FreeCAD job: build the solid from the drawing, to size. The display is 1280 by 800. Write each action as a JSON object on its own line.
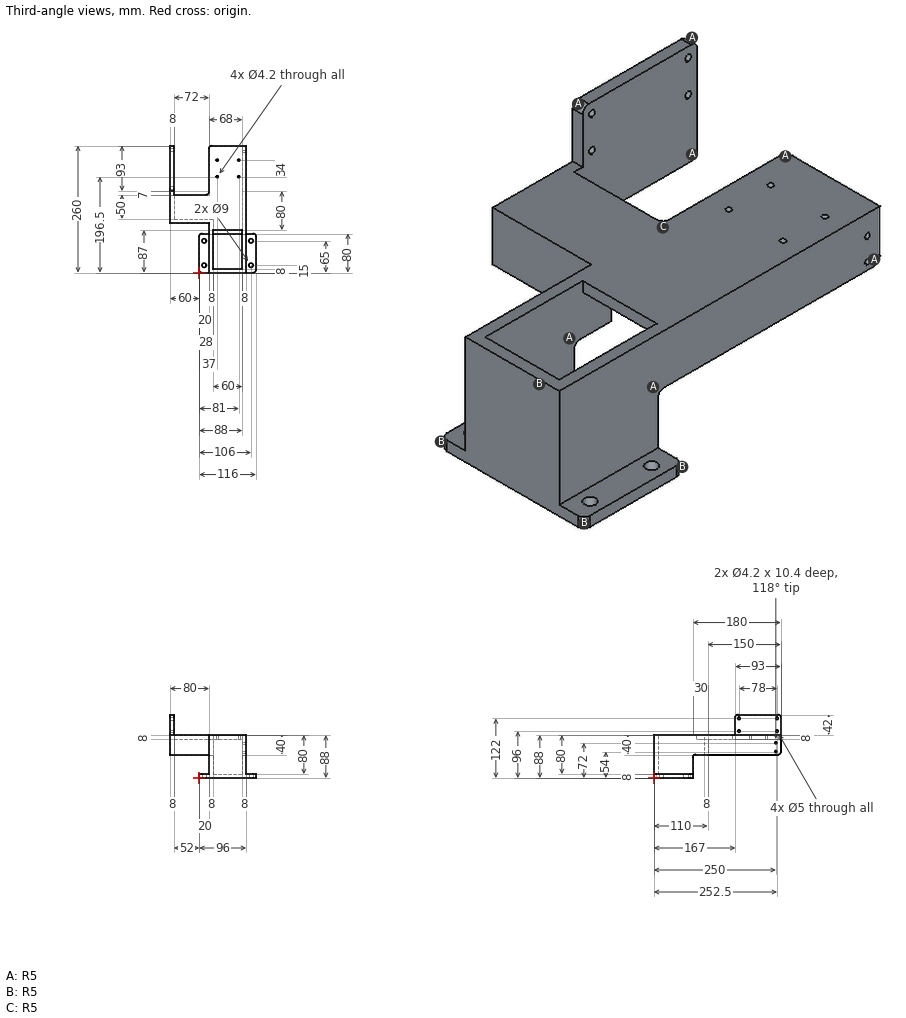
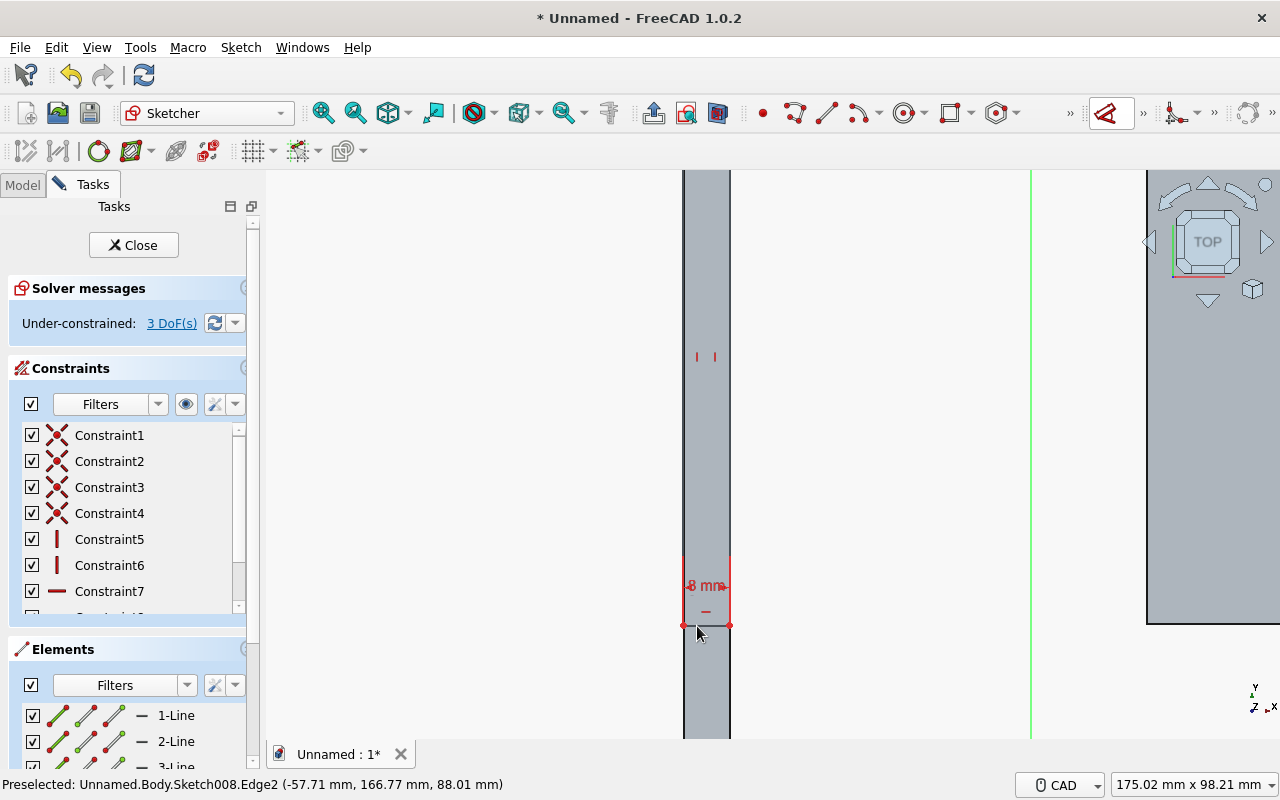
{"action": "left_click", "coordinate": [683, 249]}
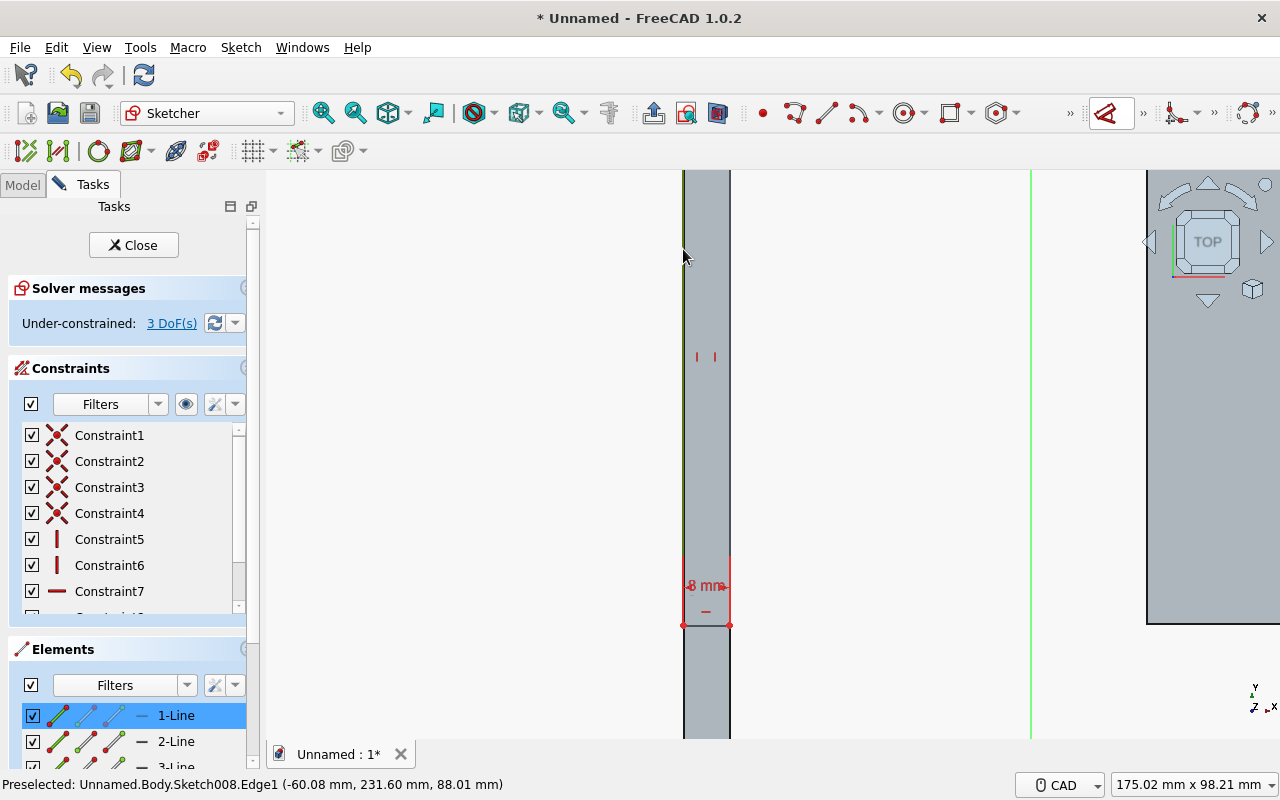
{"action": "left_click", "coordinate": [1128, 114]}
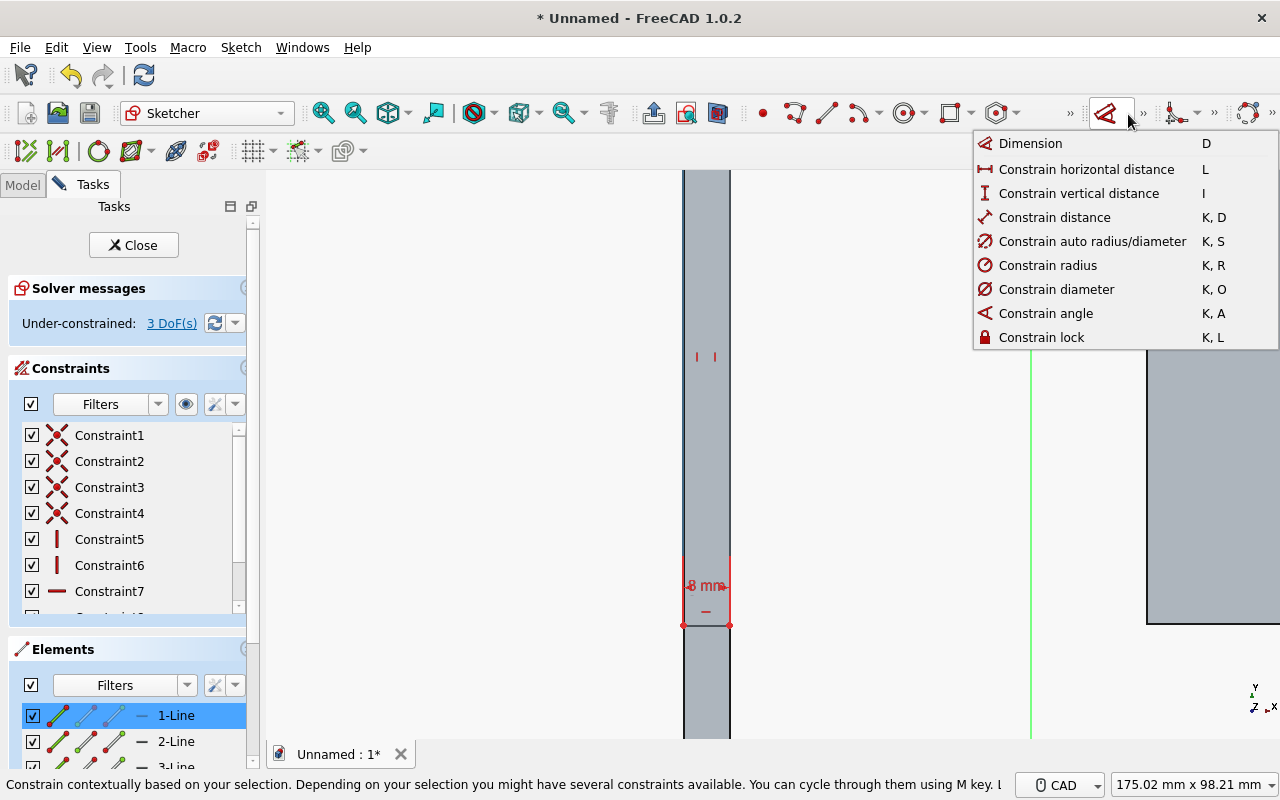
{"action": "left_click", "coordinate": [1126, 193]}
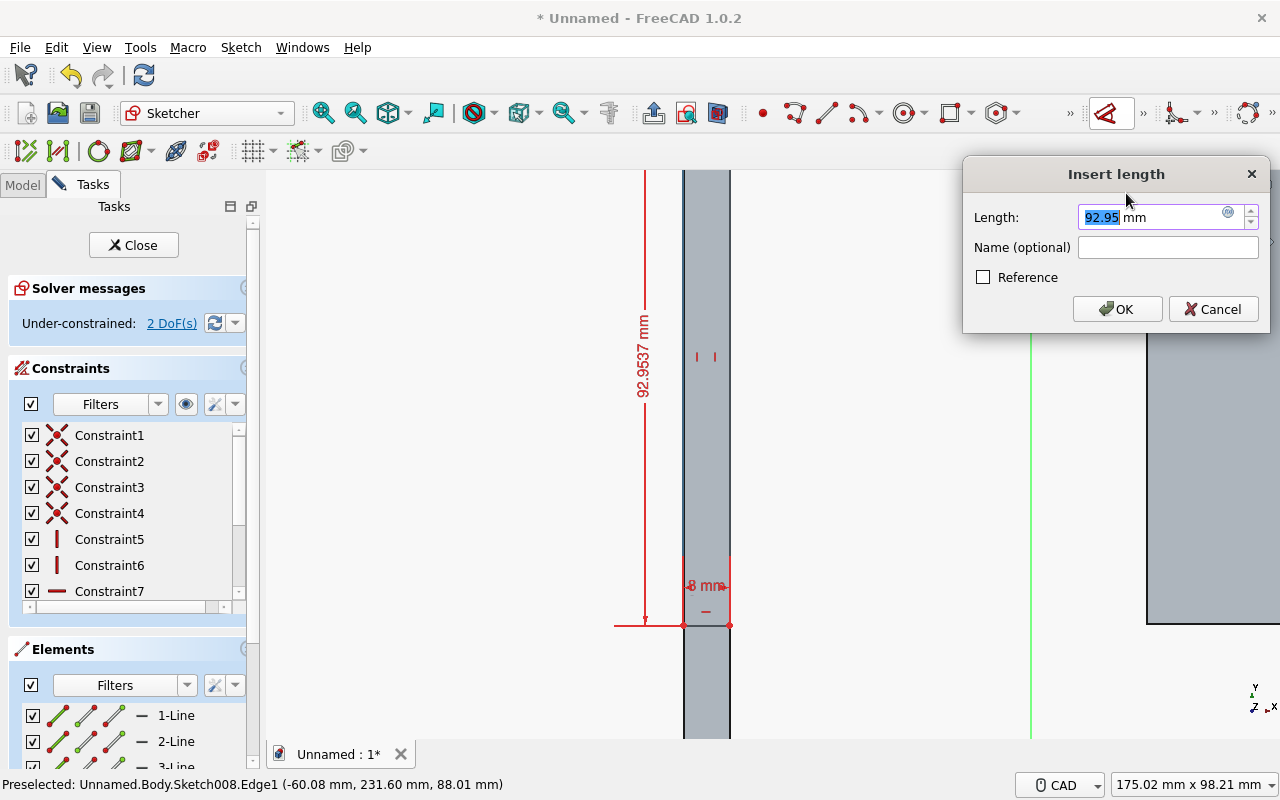
{"action": "type", "text": "93"}
{"action": "key", "text": "Return"}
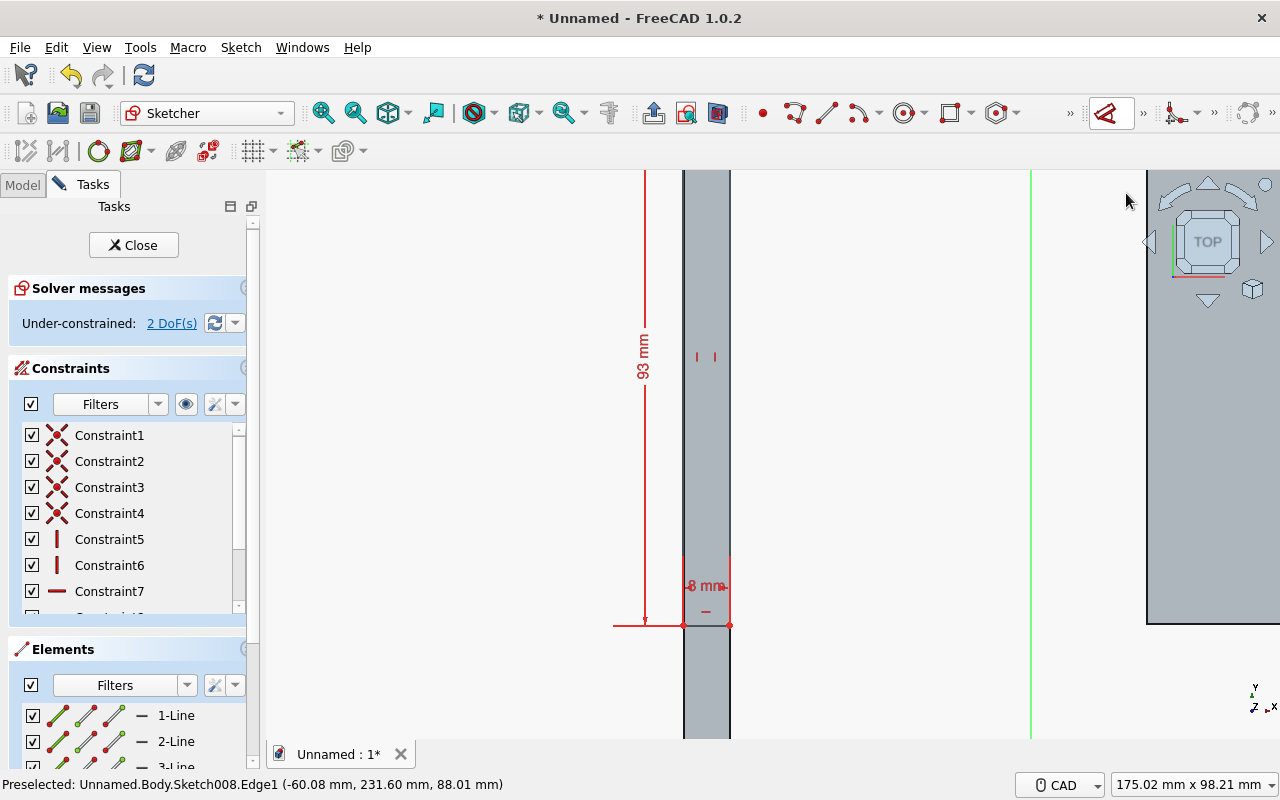
{"action": "scroll", "coordinate": [700, 657], "scroll_direction": "down", "scroll_amount": 2}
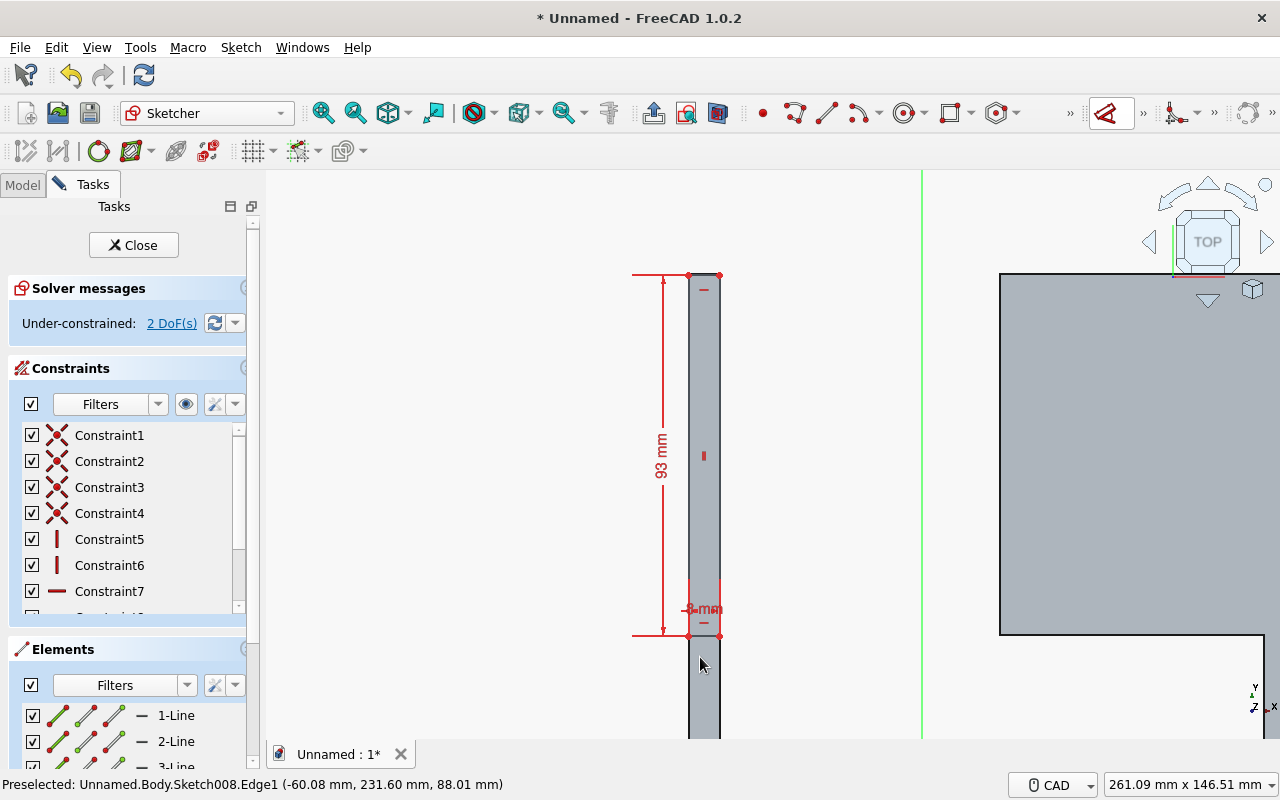
{"action": "left_click", "coordinate": [689, 275]}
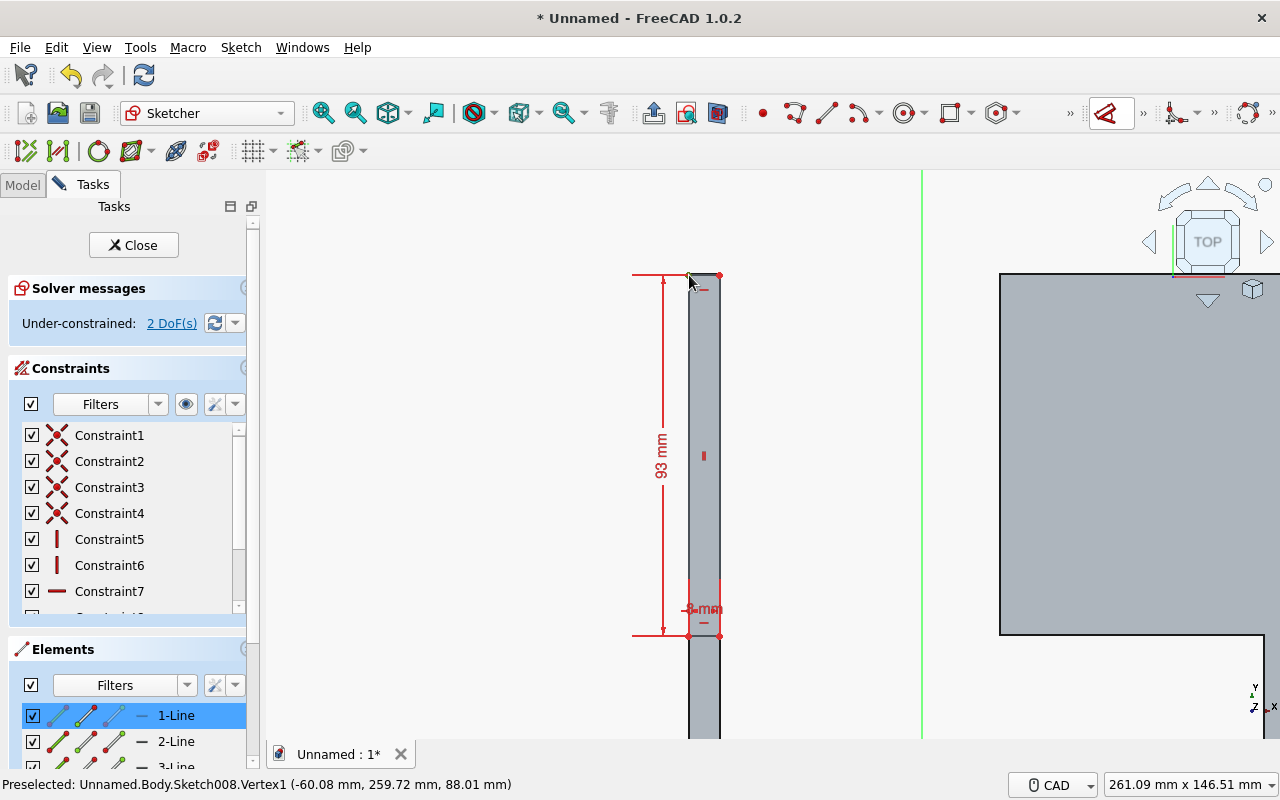
{"action": "left_click", "coordinate": [1128, 114]}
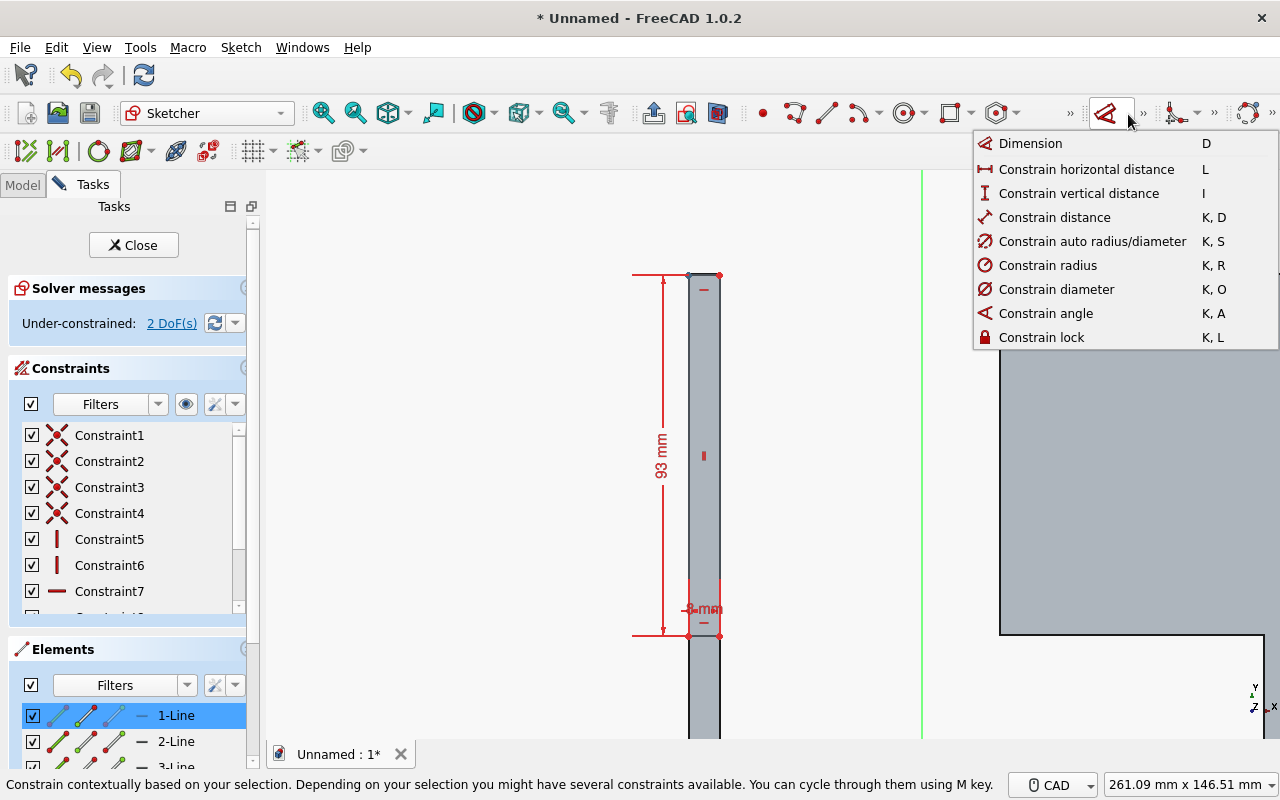
{"action": "left_click", "coordinate": [1126, 169]}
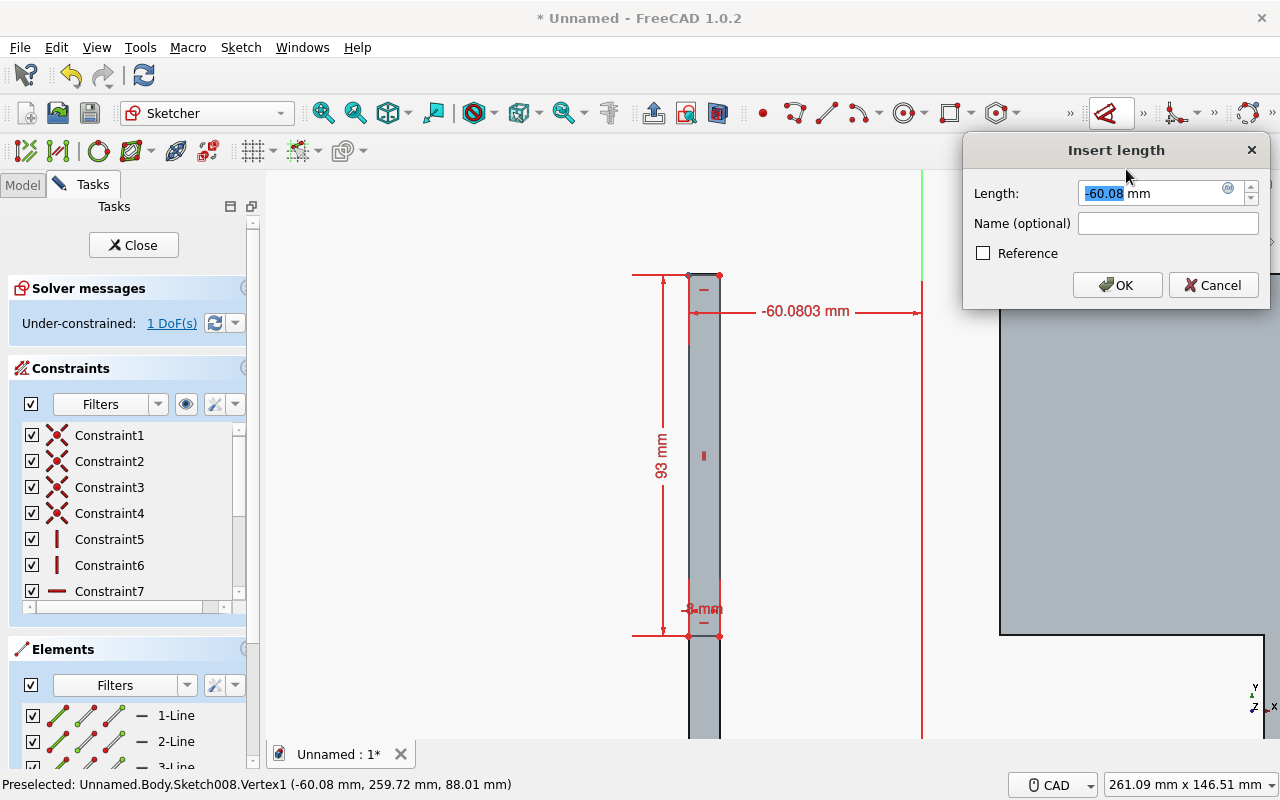
{"action": "type", "text": "-60"}
{"action": "key", "text": "Return"}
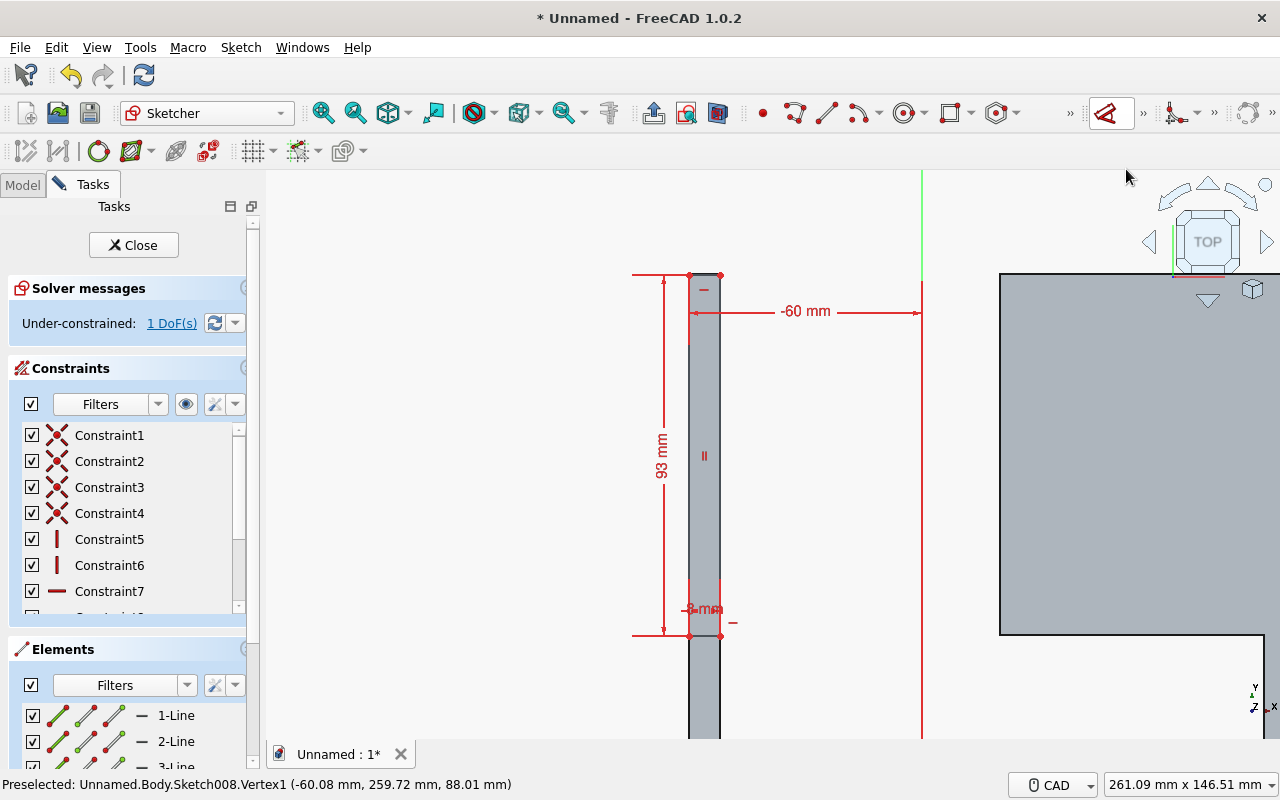
{"action": "left_click", "coordinate": [689, 275]}